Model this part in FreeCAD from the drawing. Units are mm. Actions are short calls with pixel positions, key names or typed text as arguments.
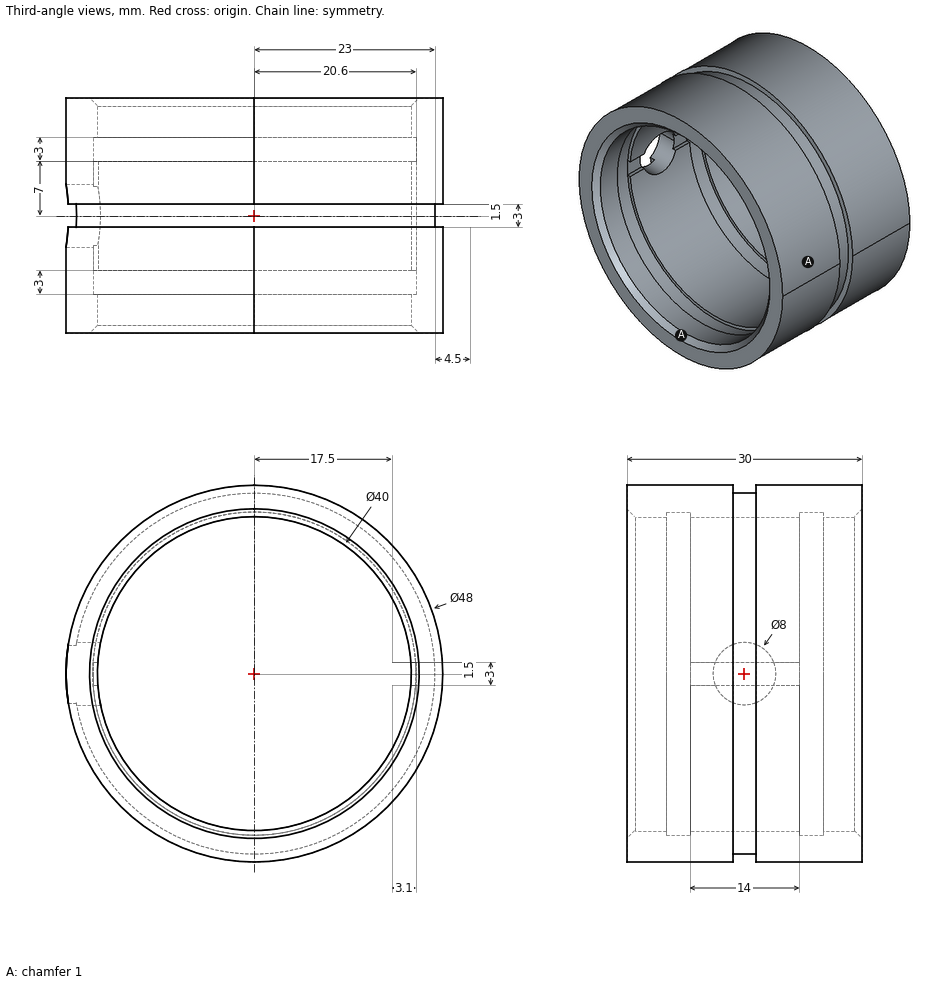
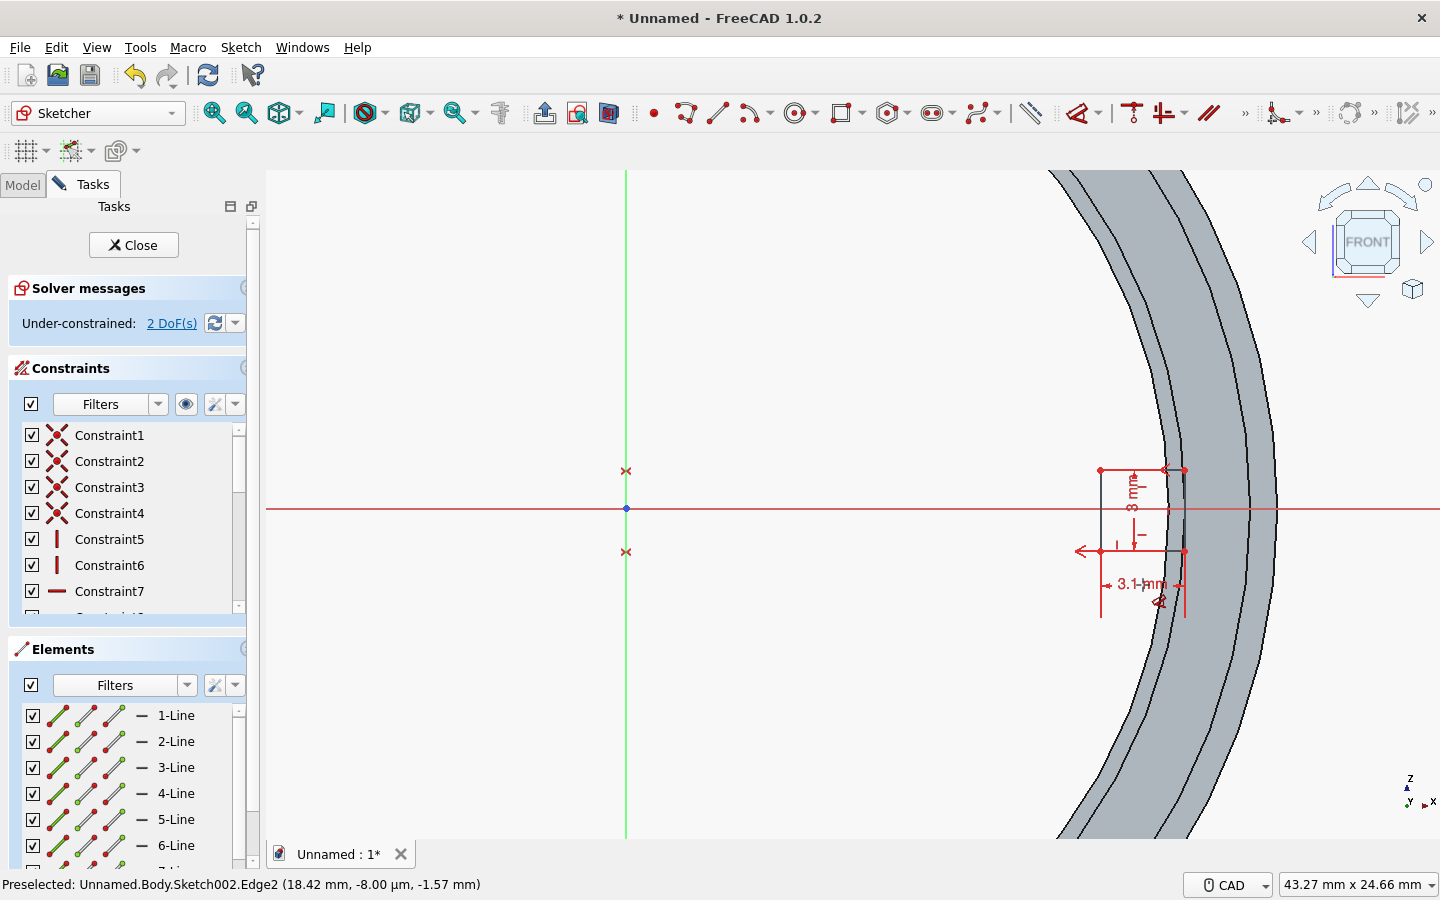
click(1101, 470)
click(592, 489)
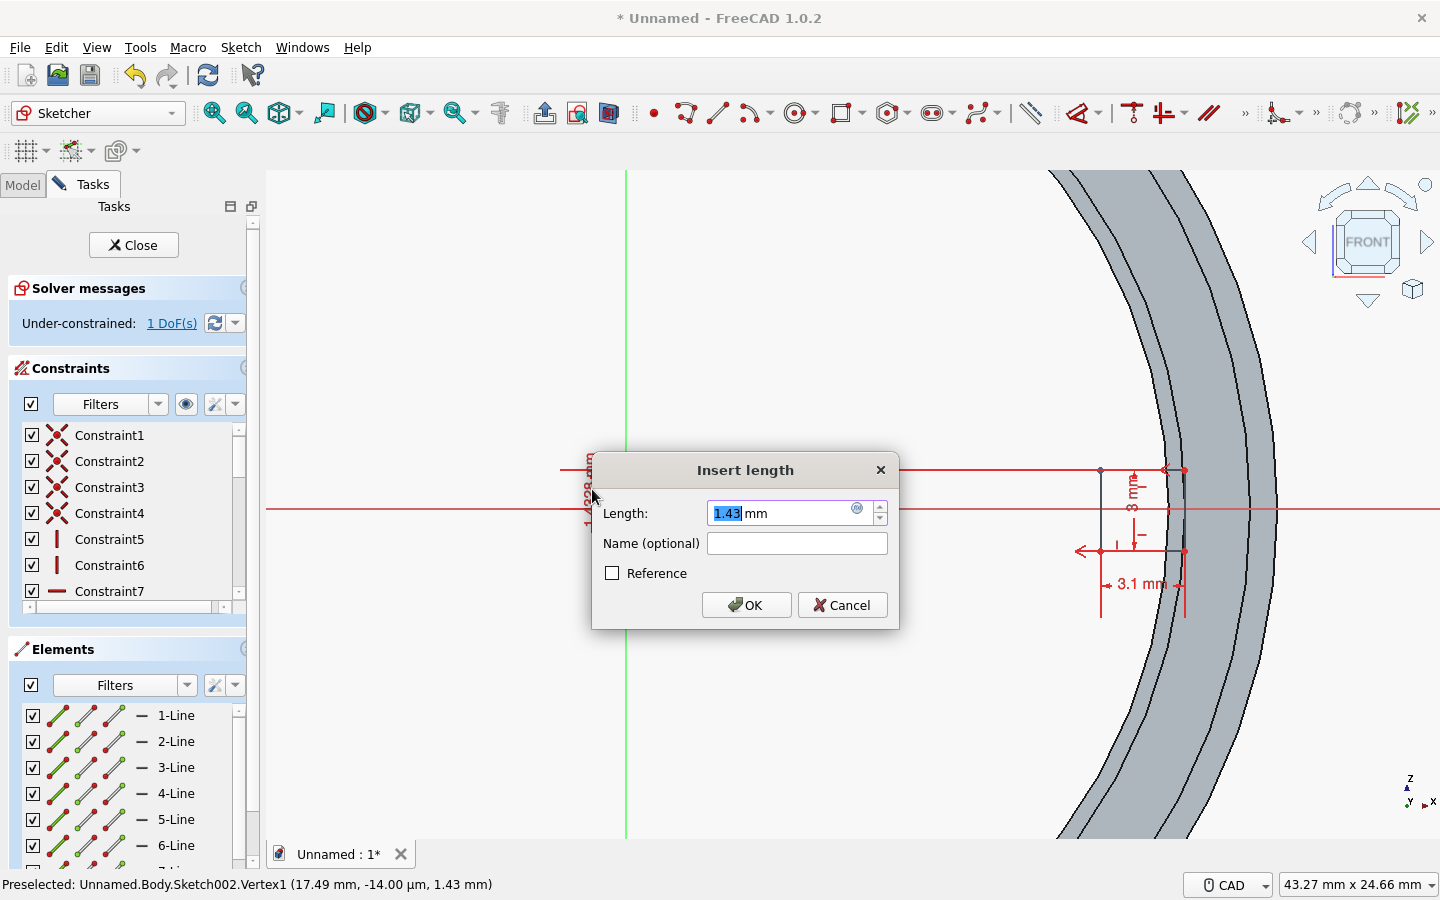
text(1.5)
key(Return)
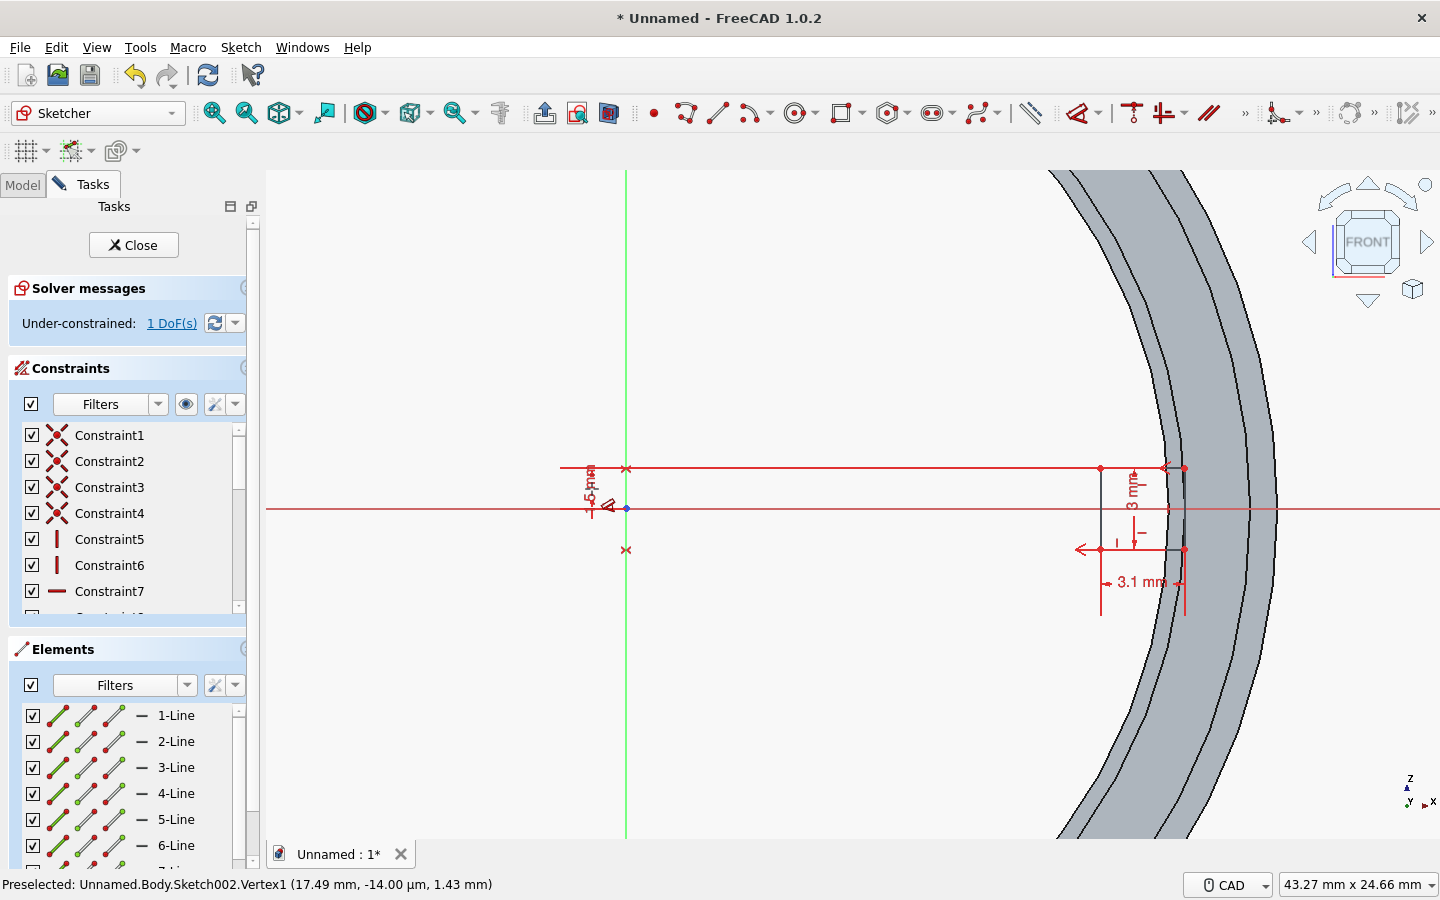
click(1101, 468)
click(863, 434)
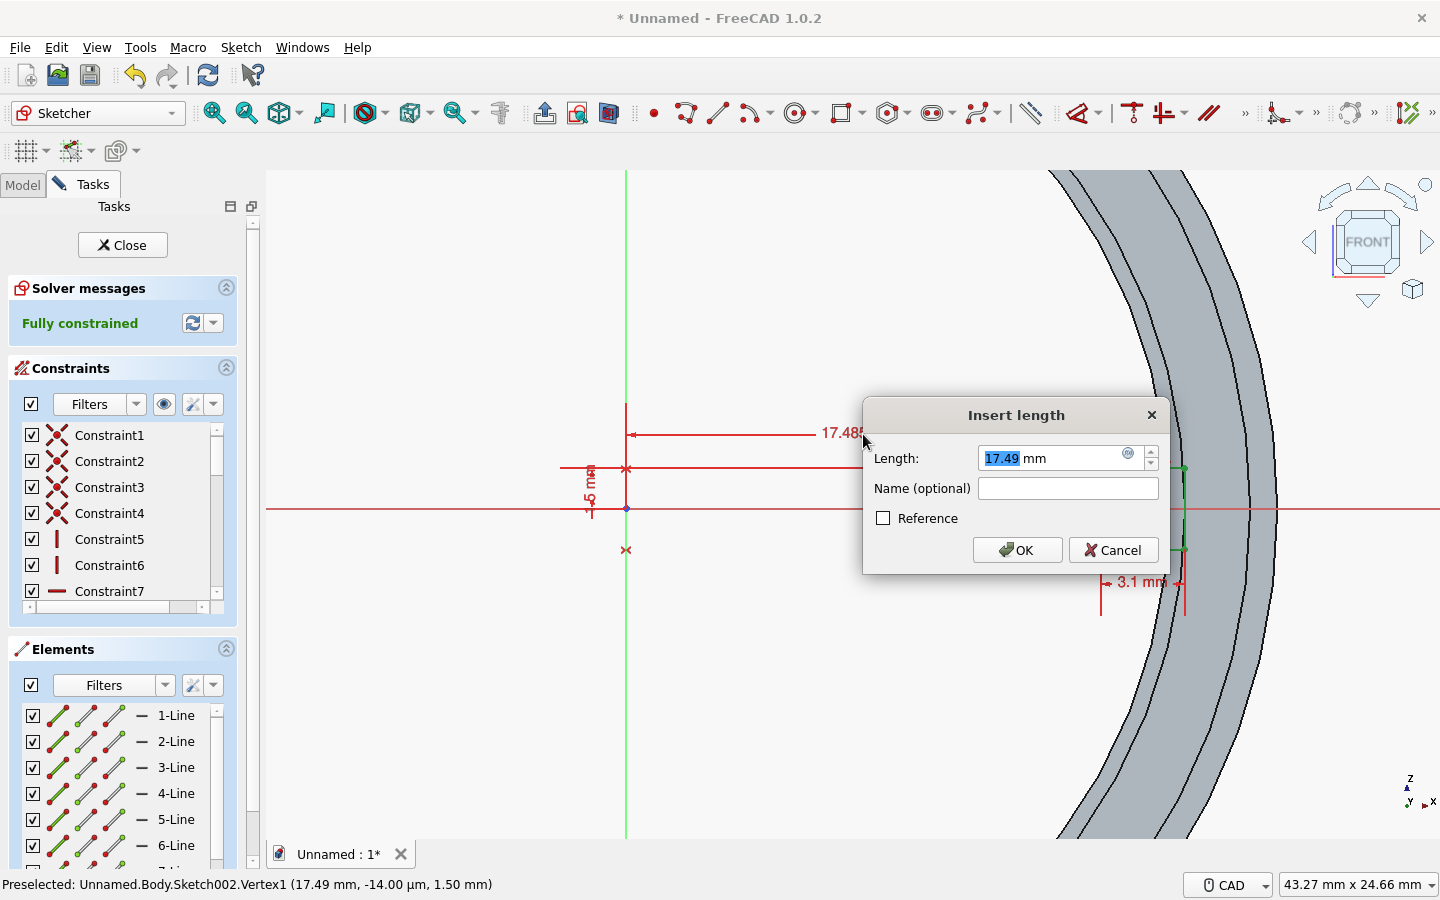
text(17.5)
key(Return)
key(Escape)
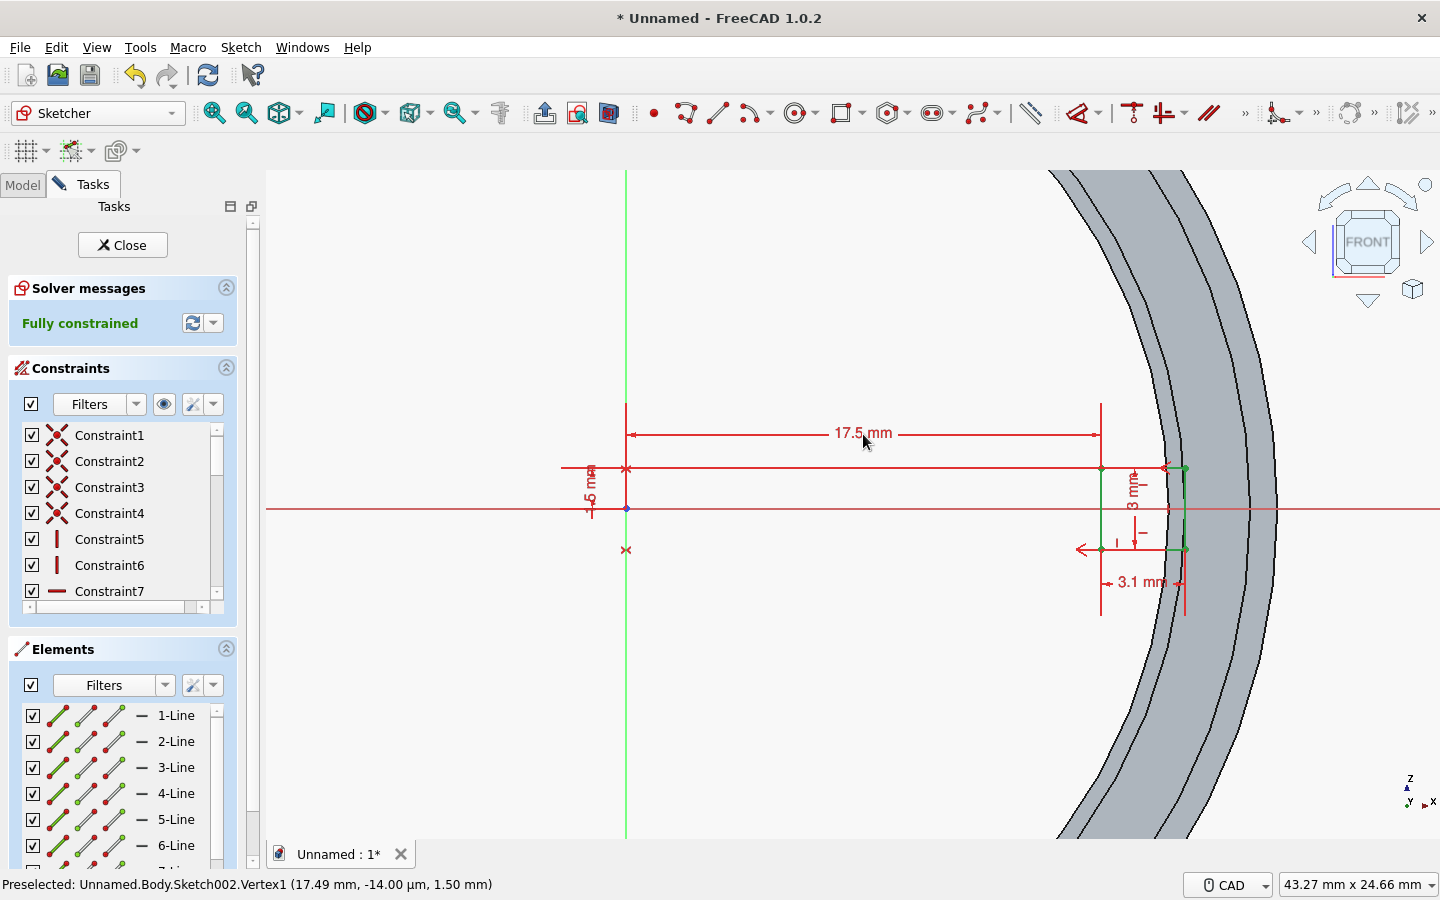
click(123, 245)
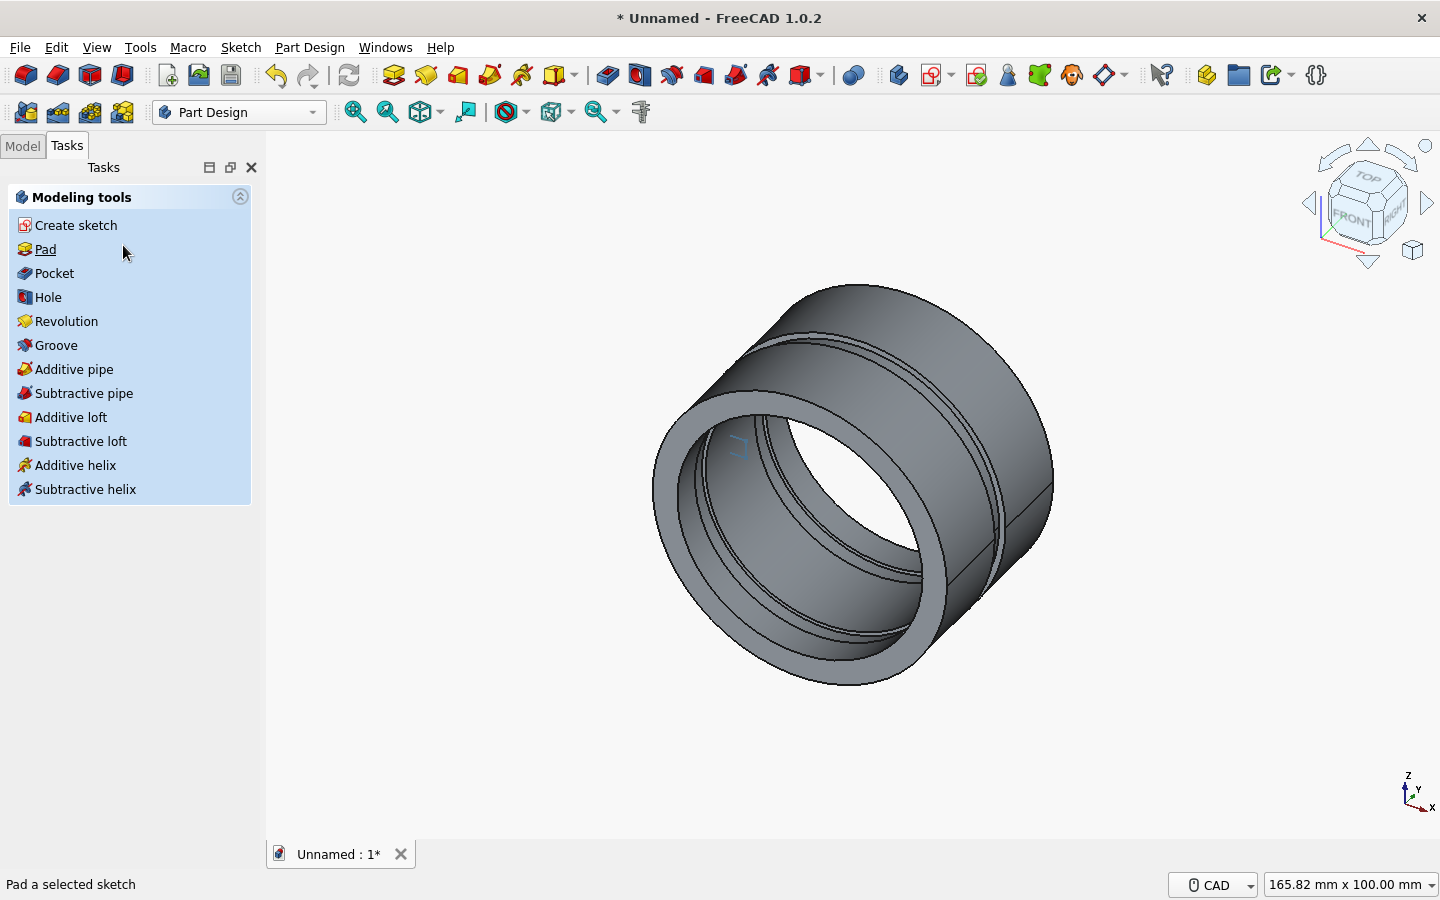
click(608, 76)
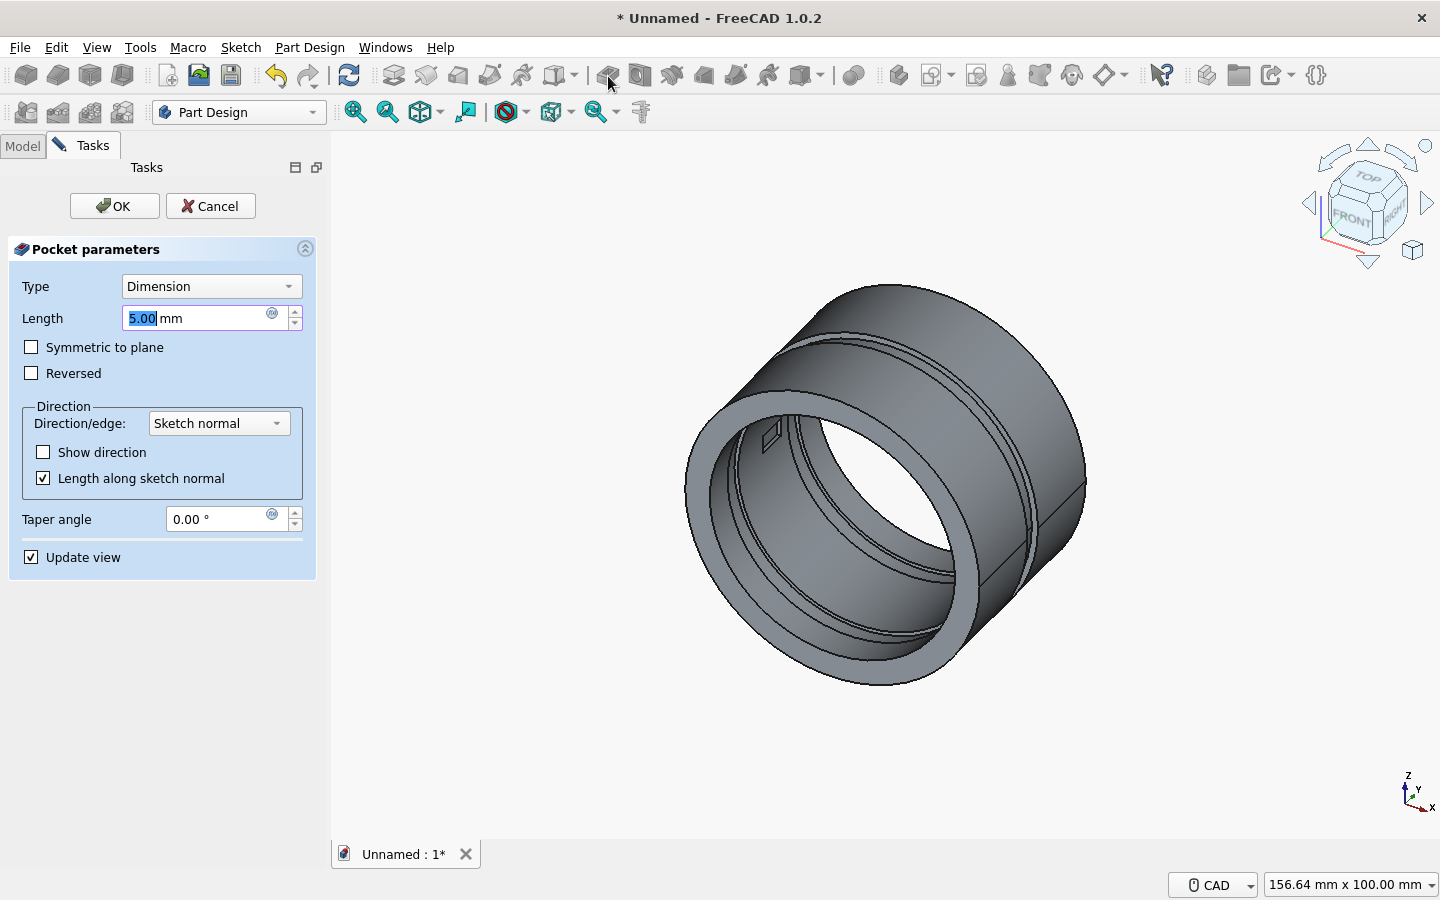
text(14)
key(Tab)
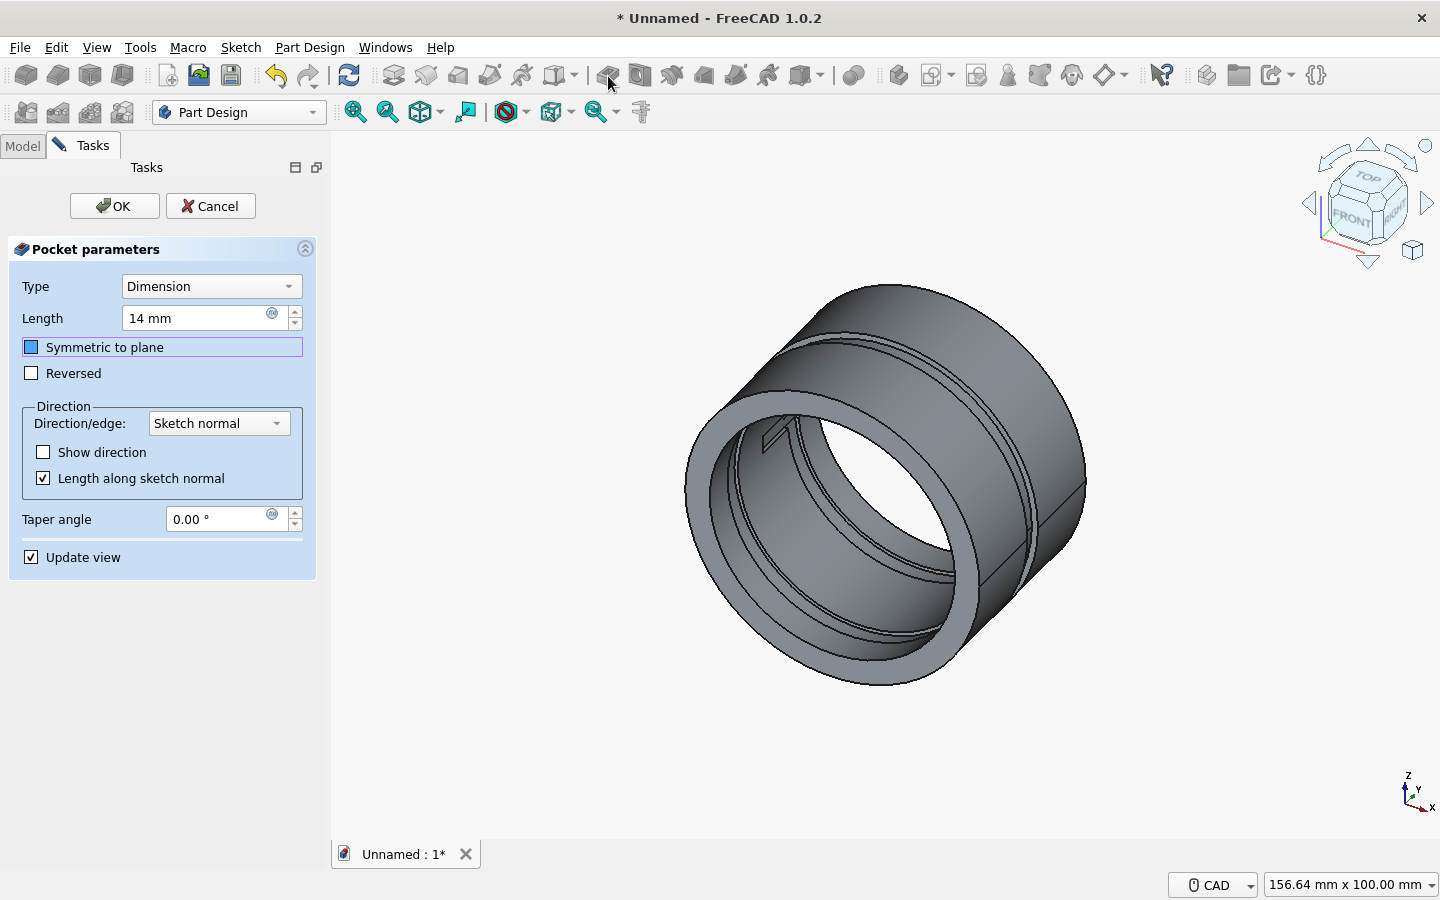
click(30, 347)